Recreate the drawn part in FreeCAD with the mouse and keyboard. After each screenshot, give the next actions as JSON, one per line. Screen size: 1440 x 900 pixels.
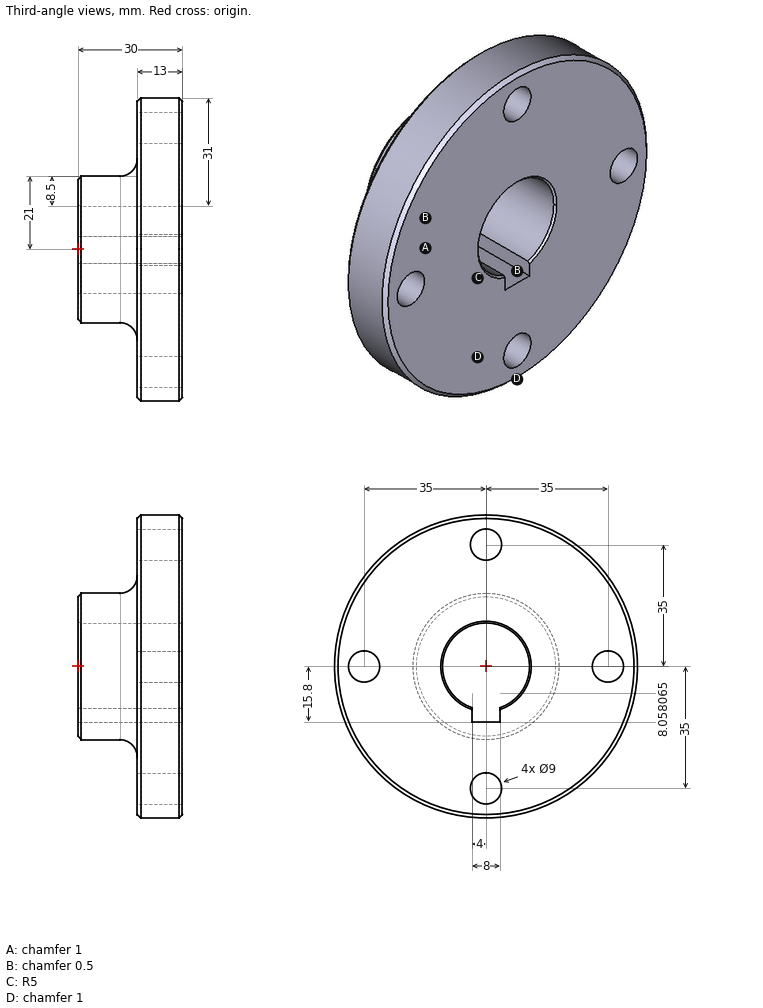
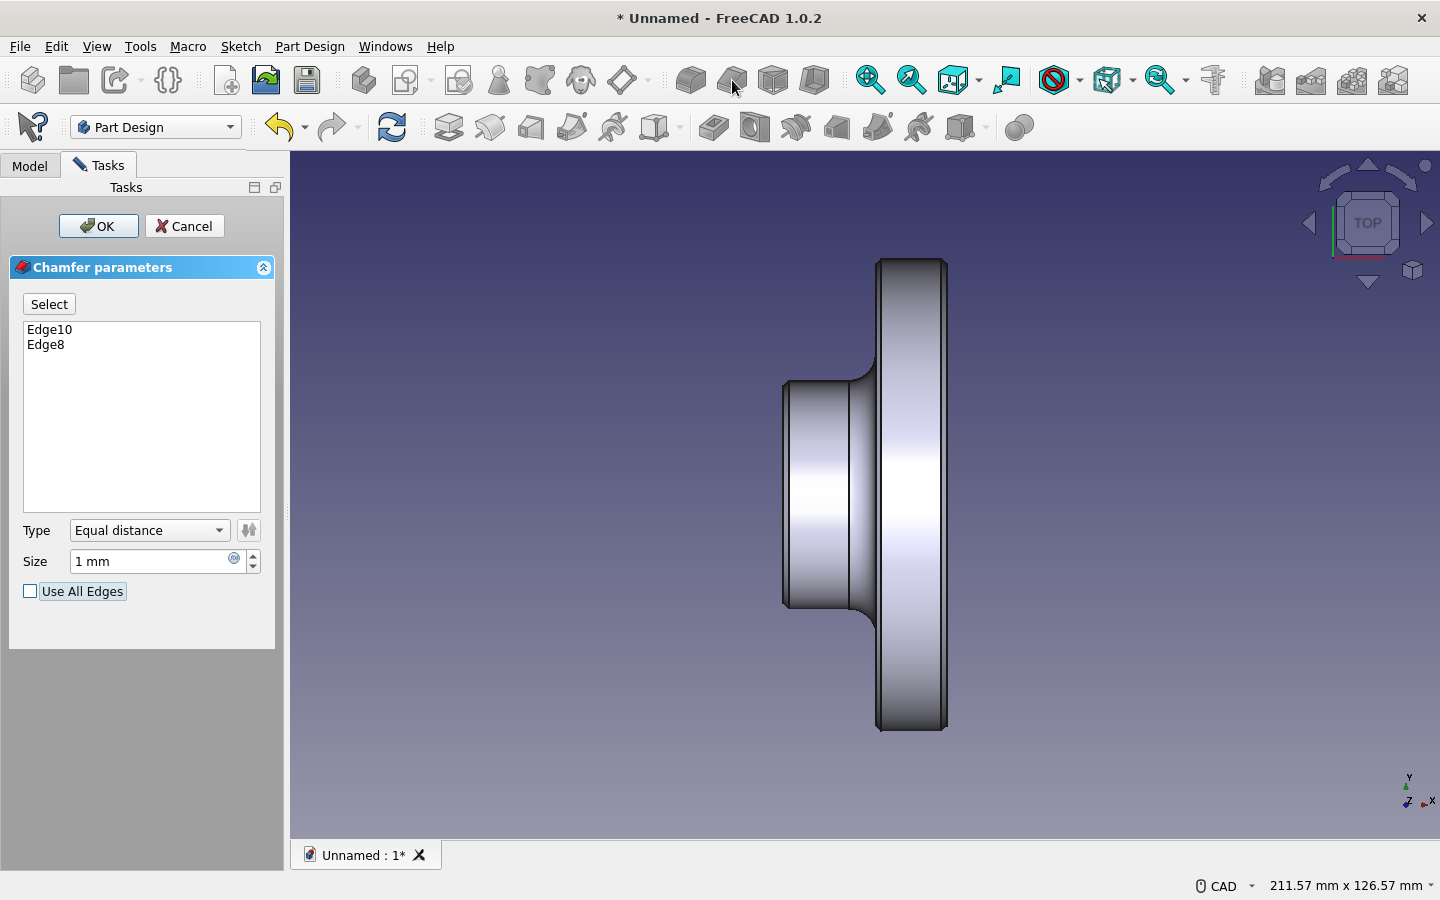
{"action": "left_click", "coordinate": [99, 226]}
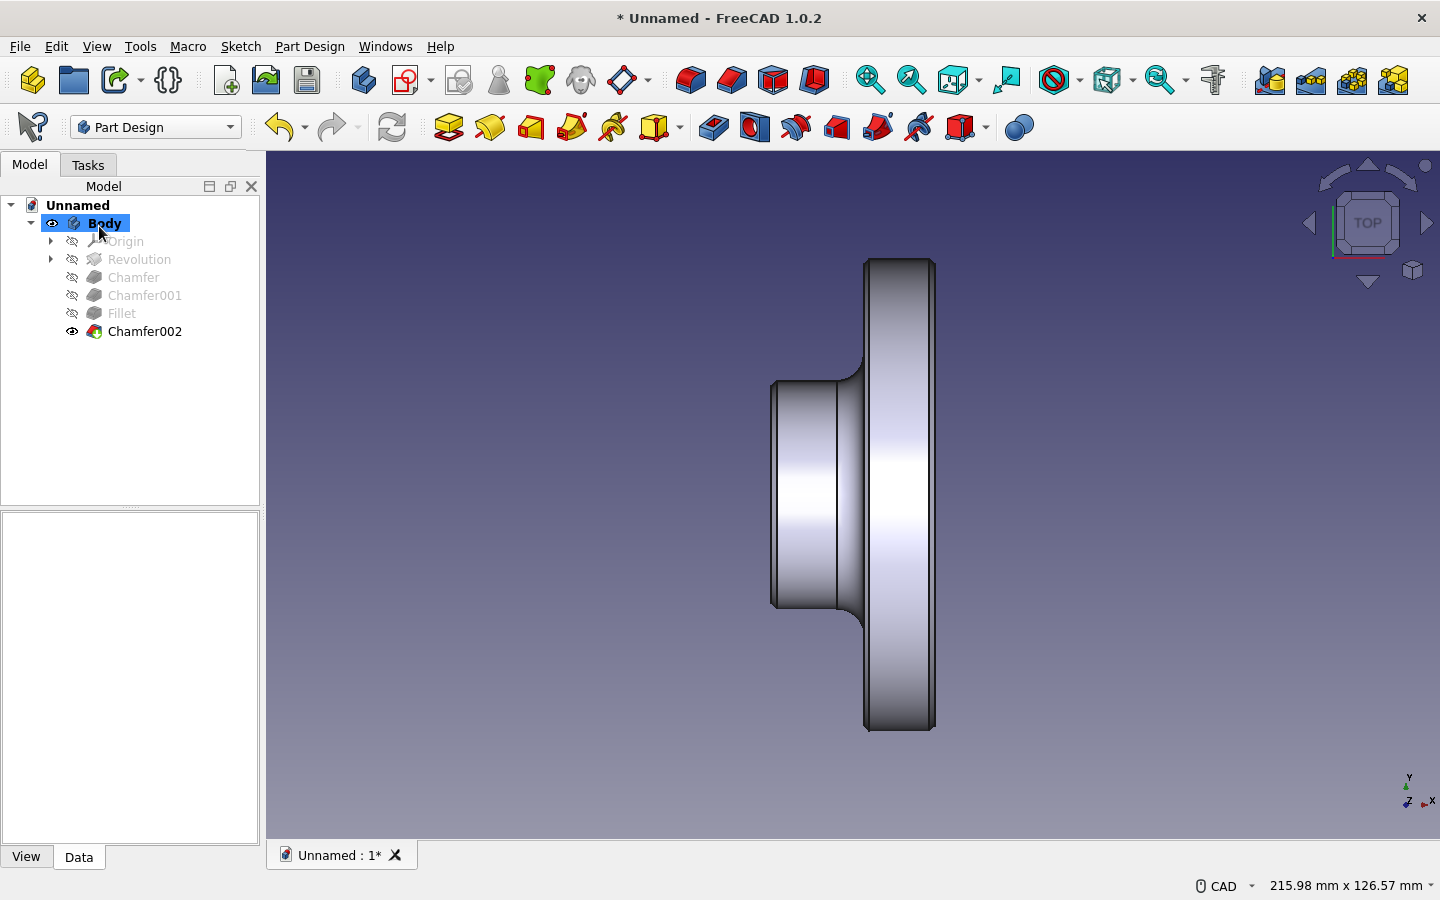
{"action": "key", "text": "6"}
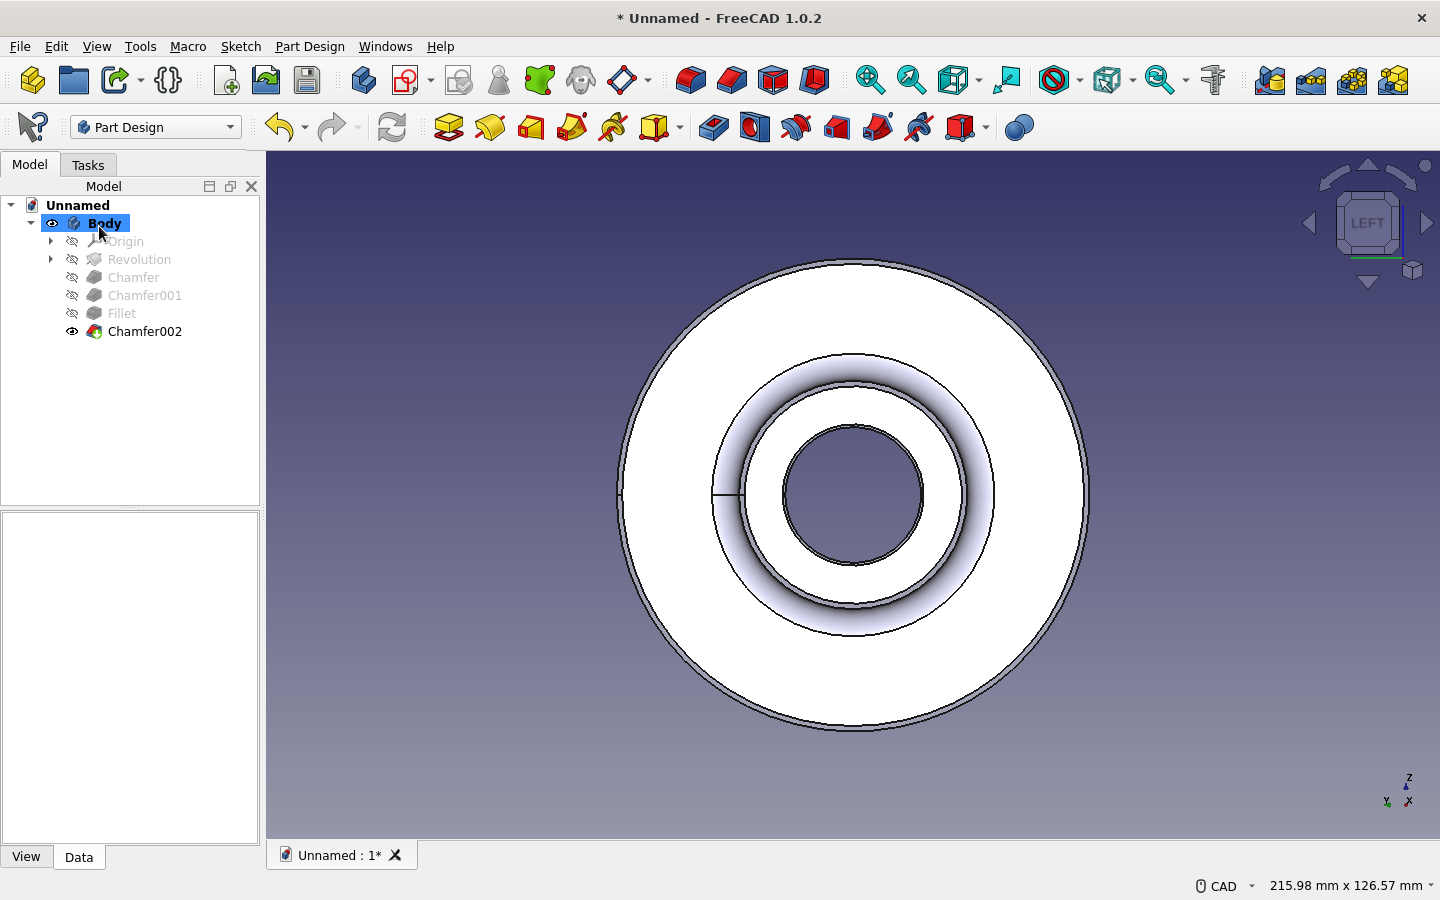
{"action": "left_click", "coordinate": [985, 626]}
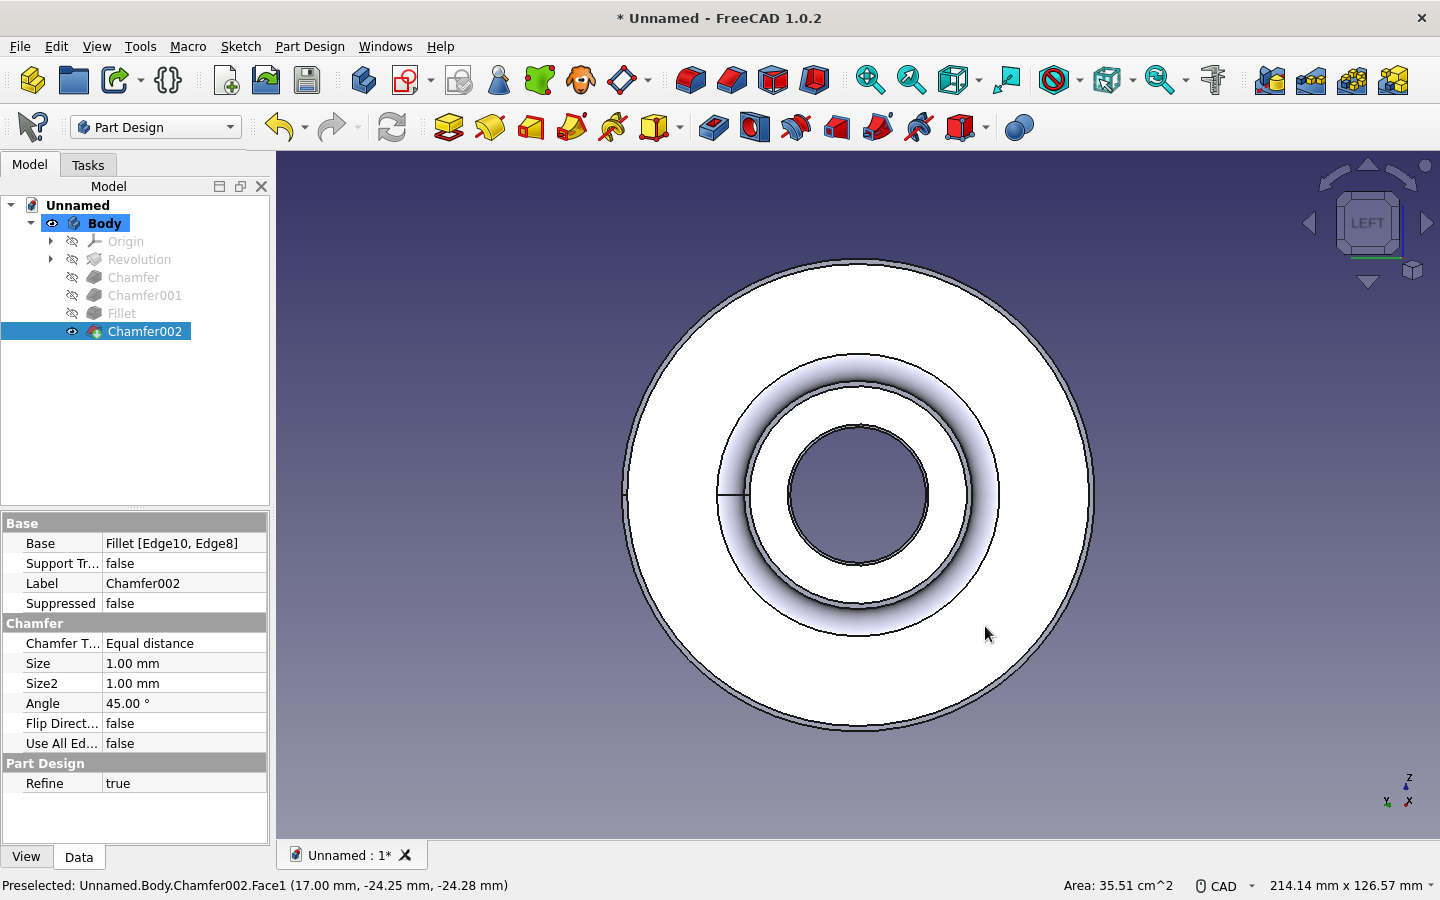
{"action": "left_click", "coordinate": [404, 80]}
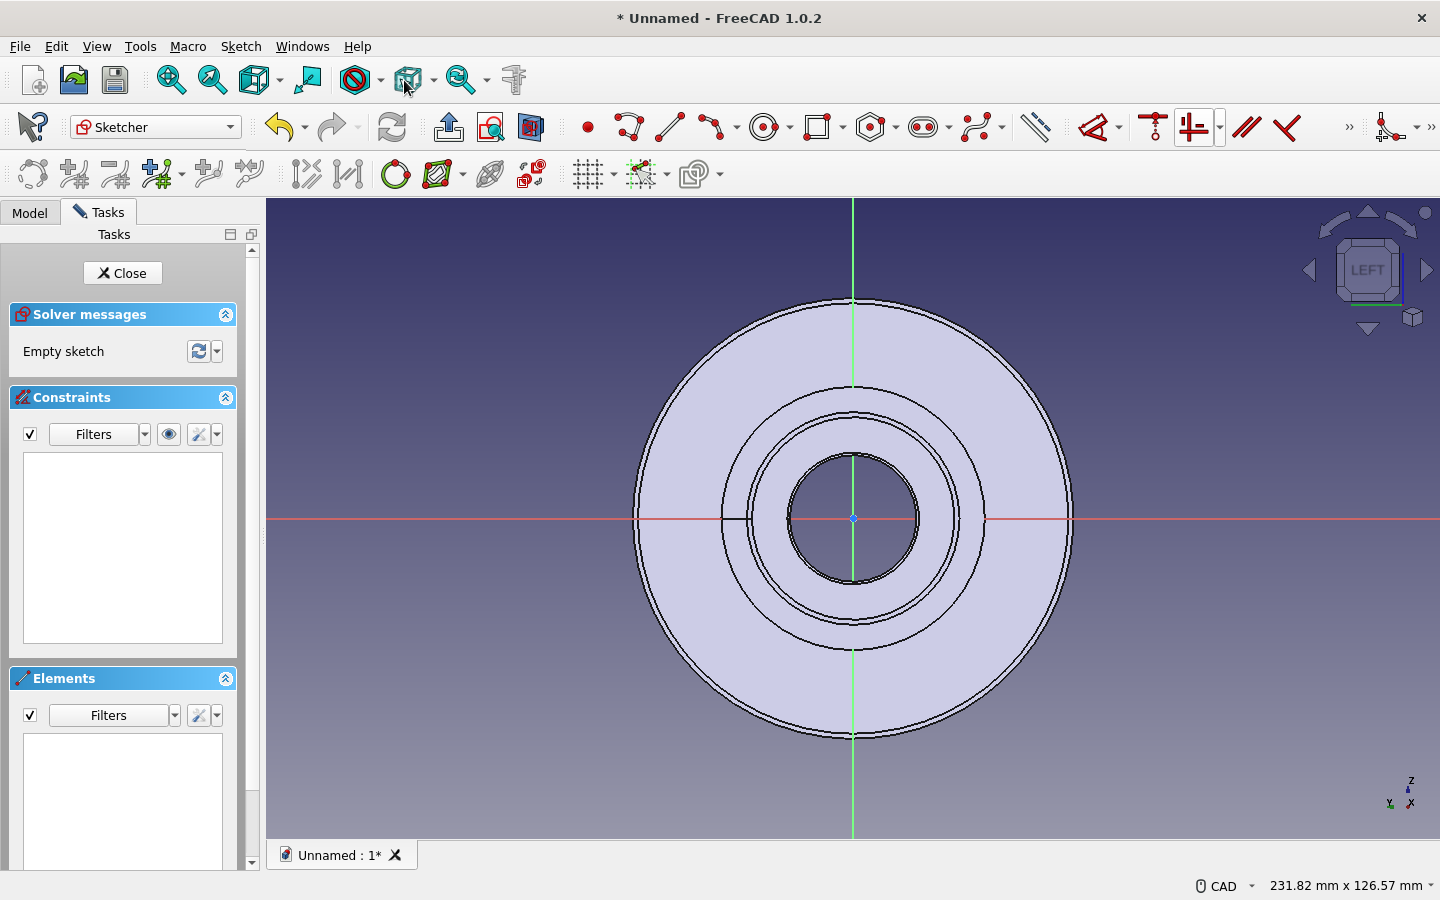
{"action": "left_click", "coordinate": [531, 128]}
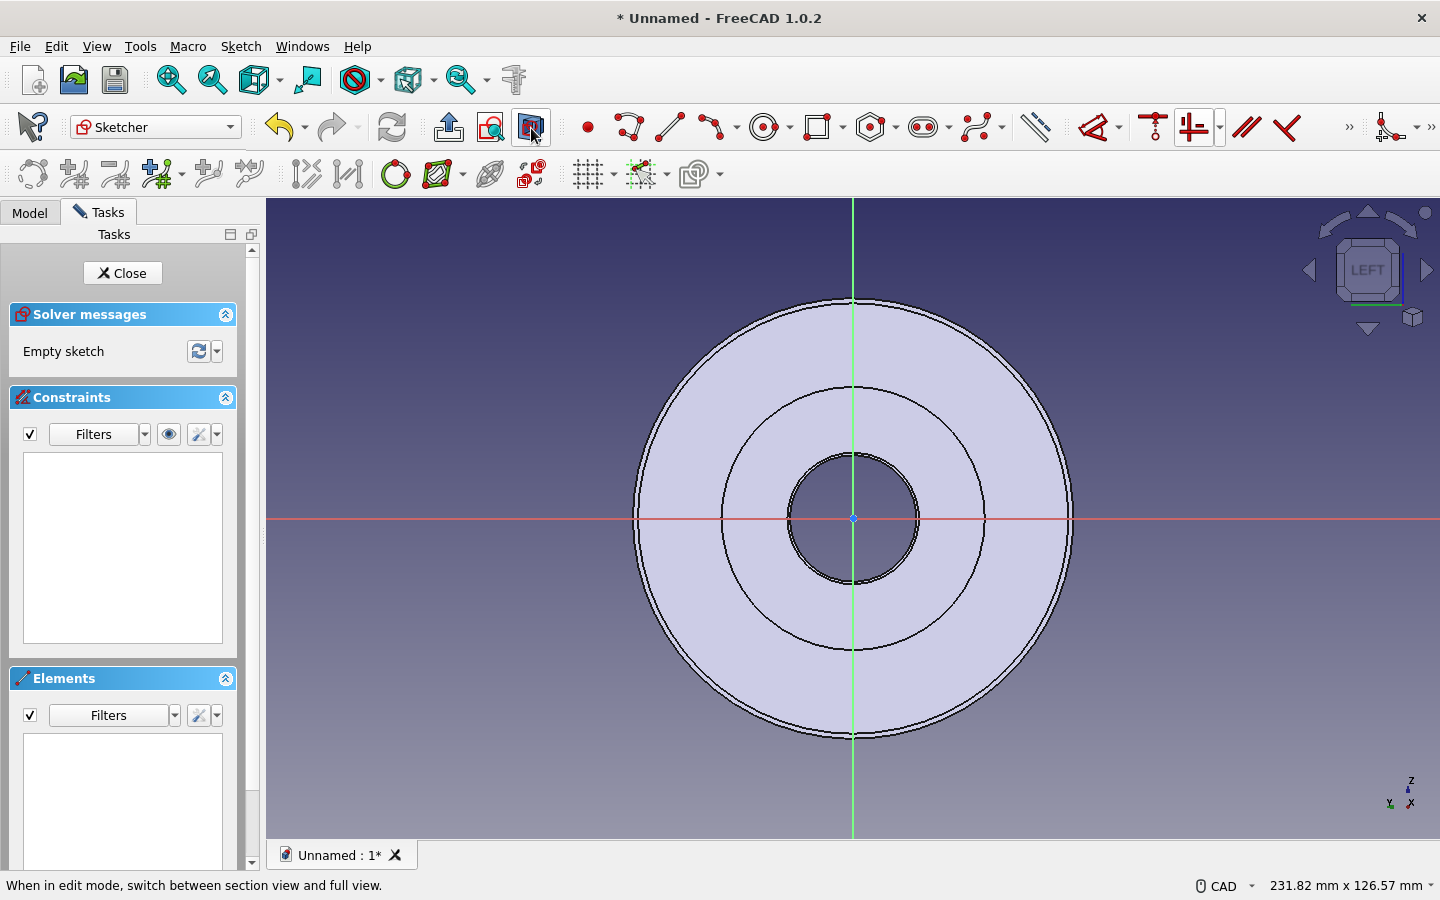
{"action": "left_click", "coordinate": [764, 128]}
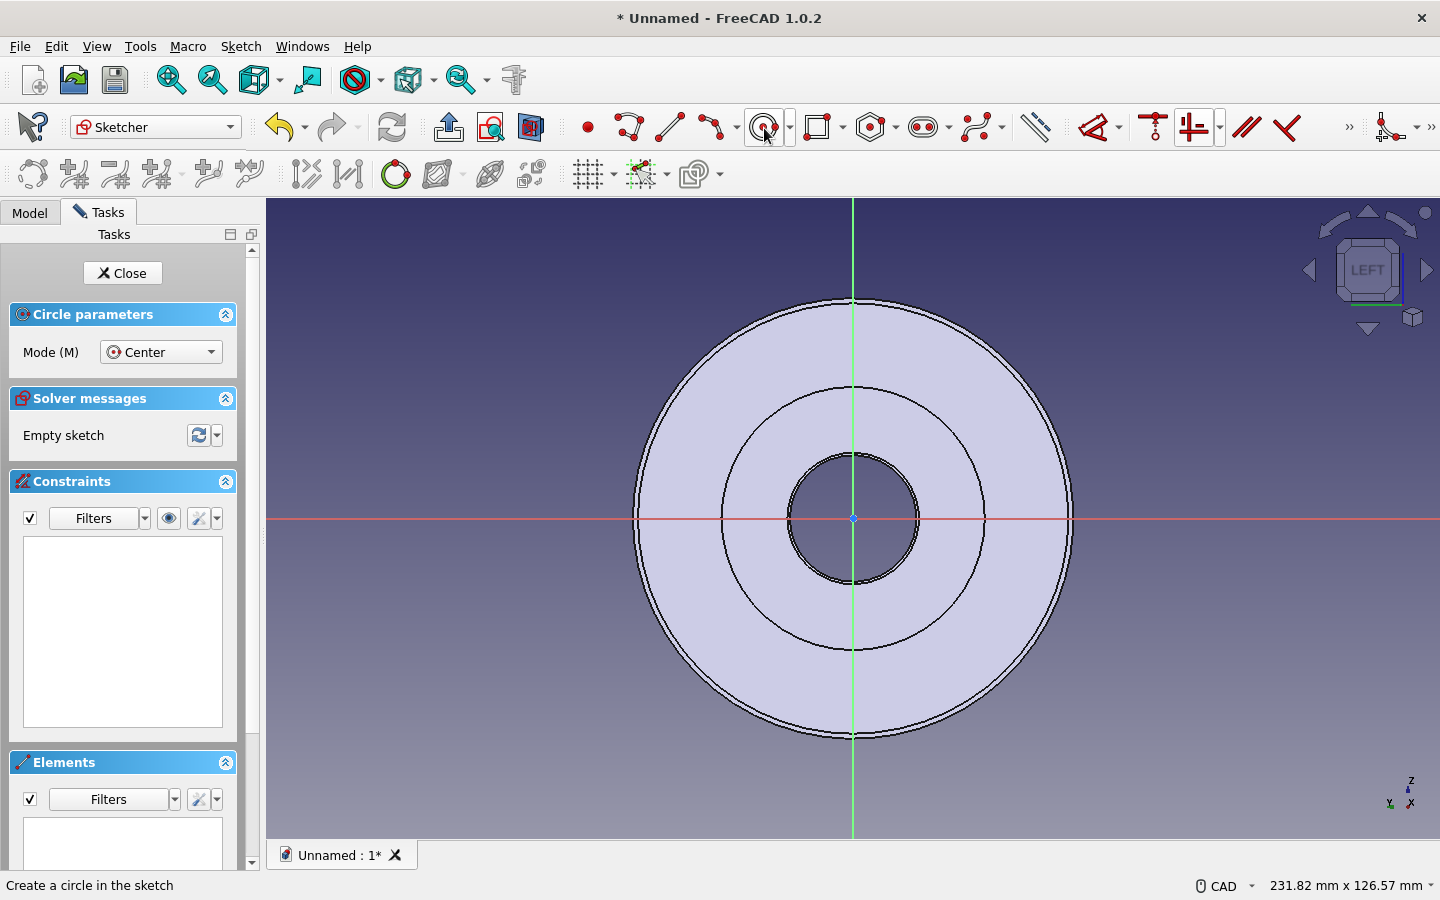
{"action": "left_click", "coordinate": [853, 696]}
{"action": "mouse_move", "coordinate": [869, 680]}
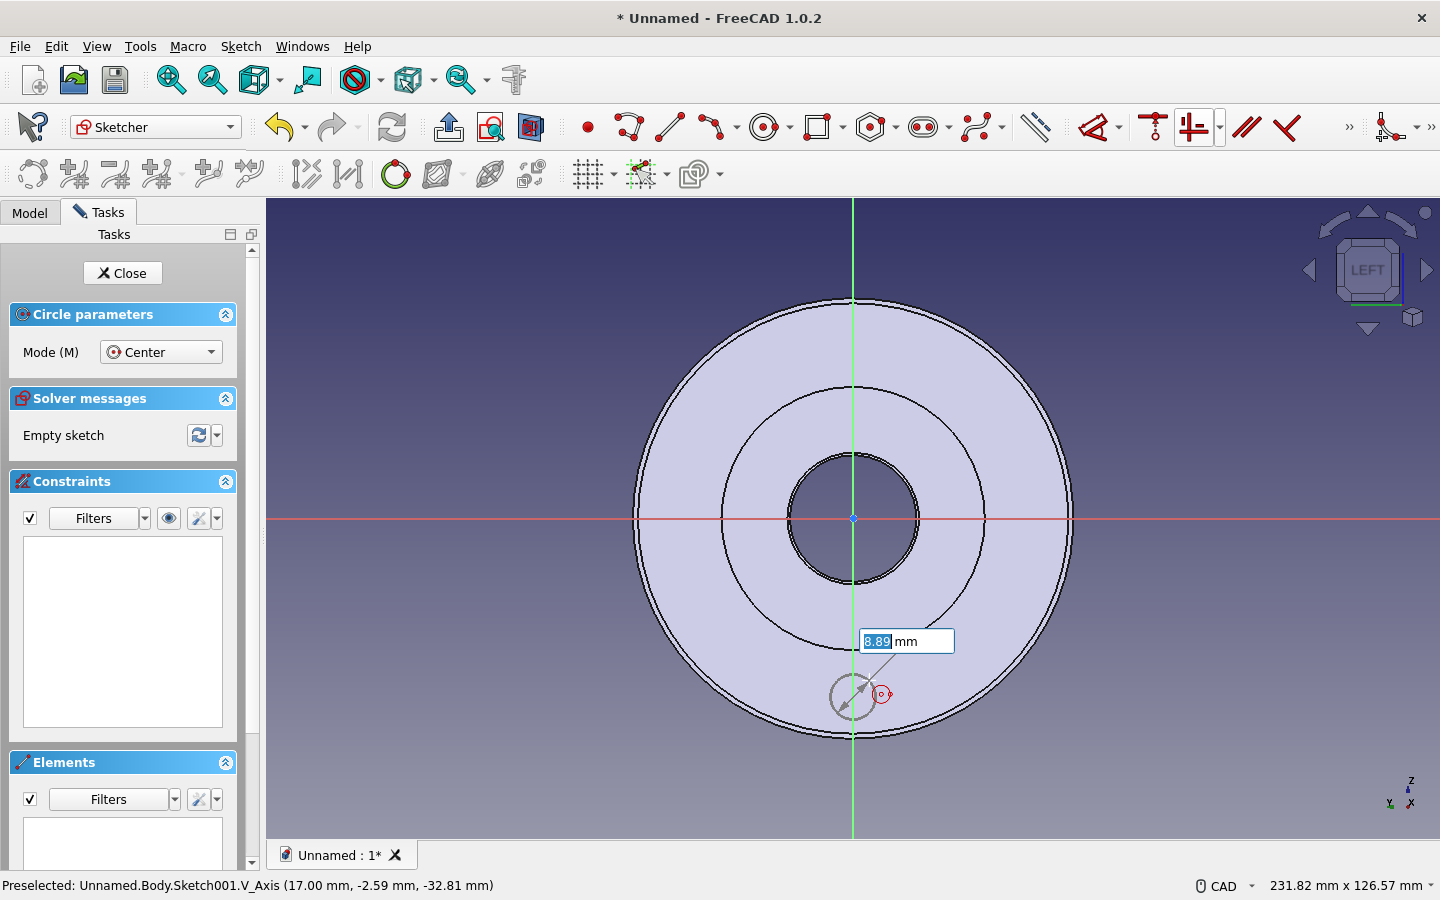
{"action": "type", "text": "9"}
{"action": "key", "text": "Return"}